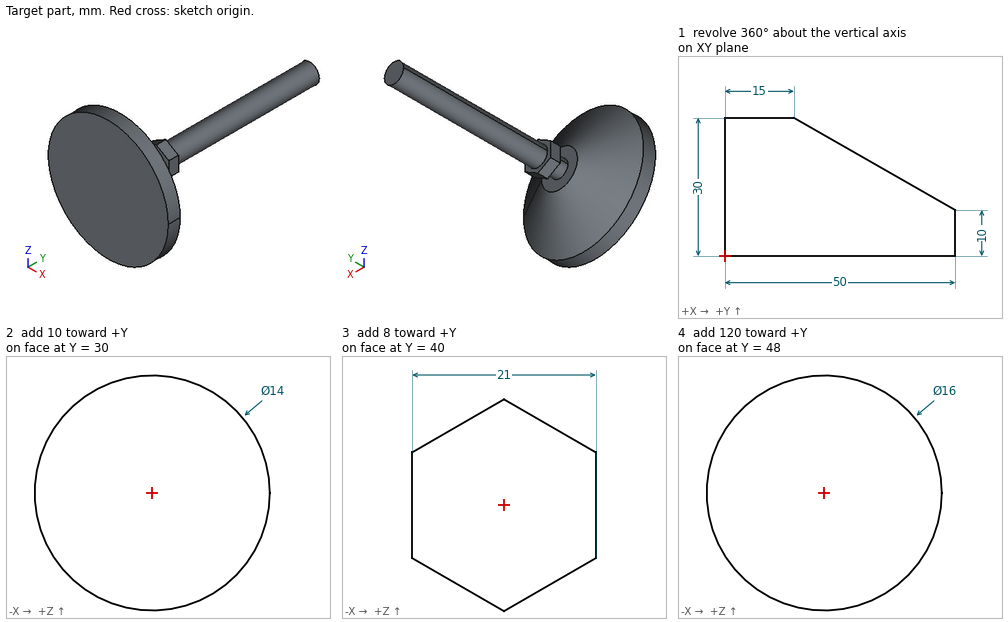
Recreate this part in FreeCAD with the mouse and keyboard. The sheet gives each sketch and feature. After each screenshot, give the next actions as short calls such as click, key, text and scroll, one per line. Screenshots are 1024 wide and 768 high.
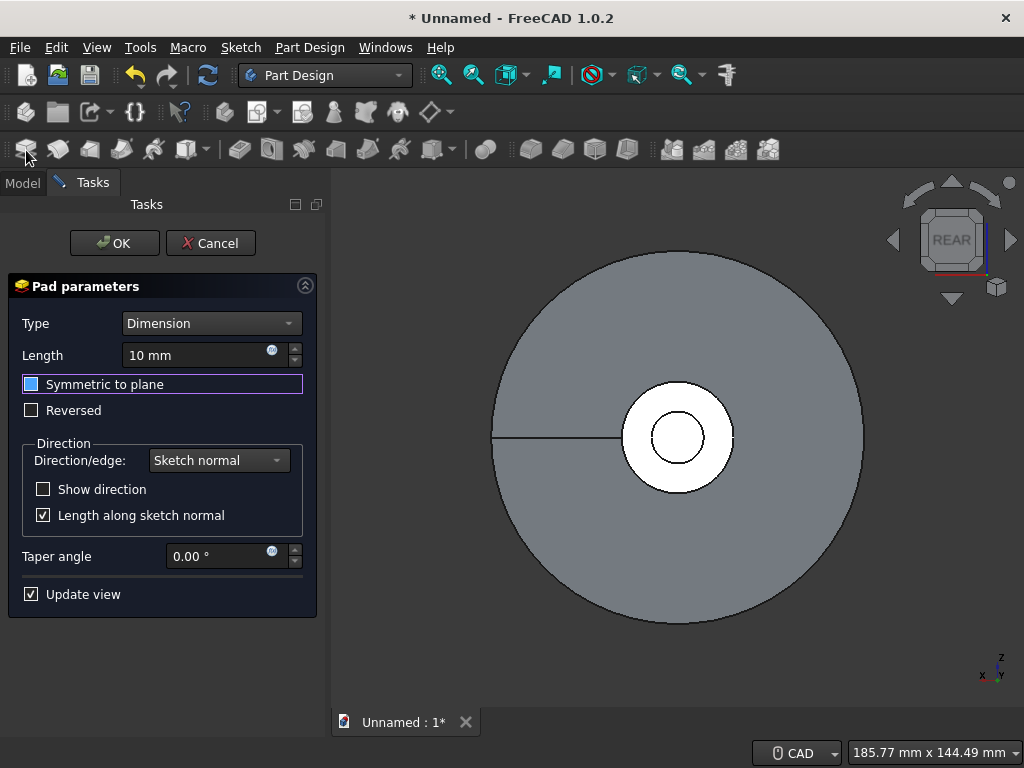
click(115, 243)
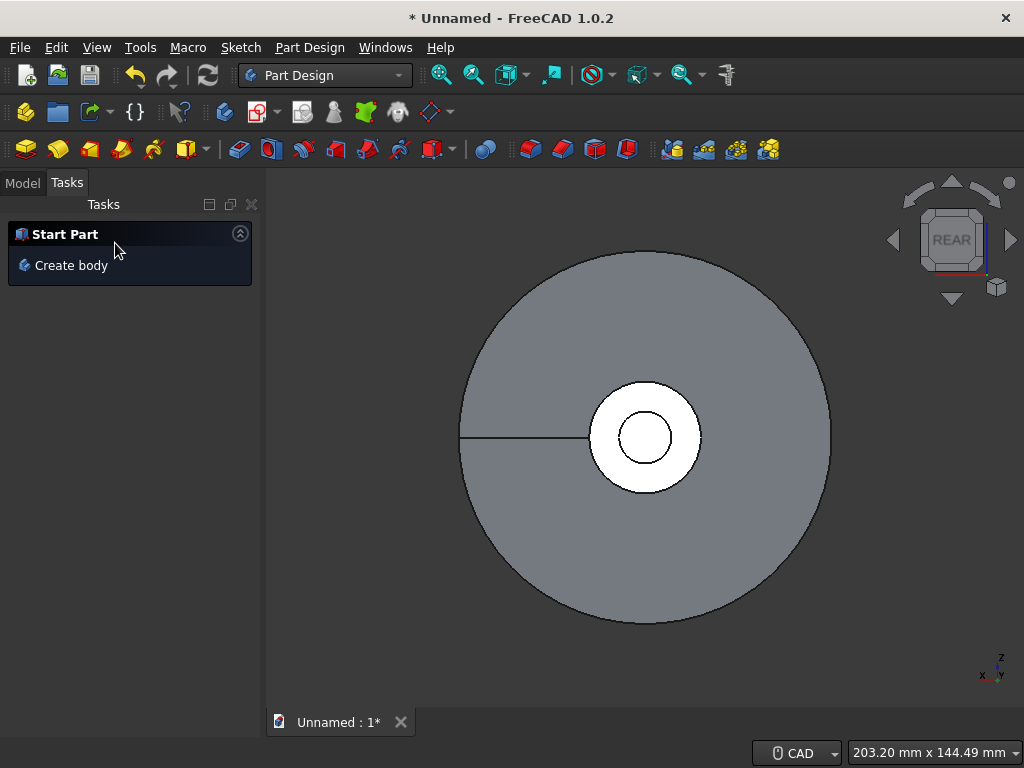
click(645, 436)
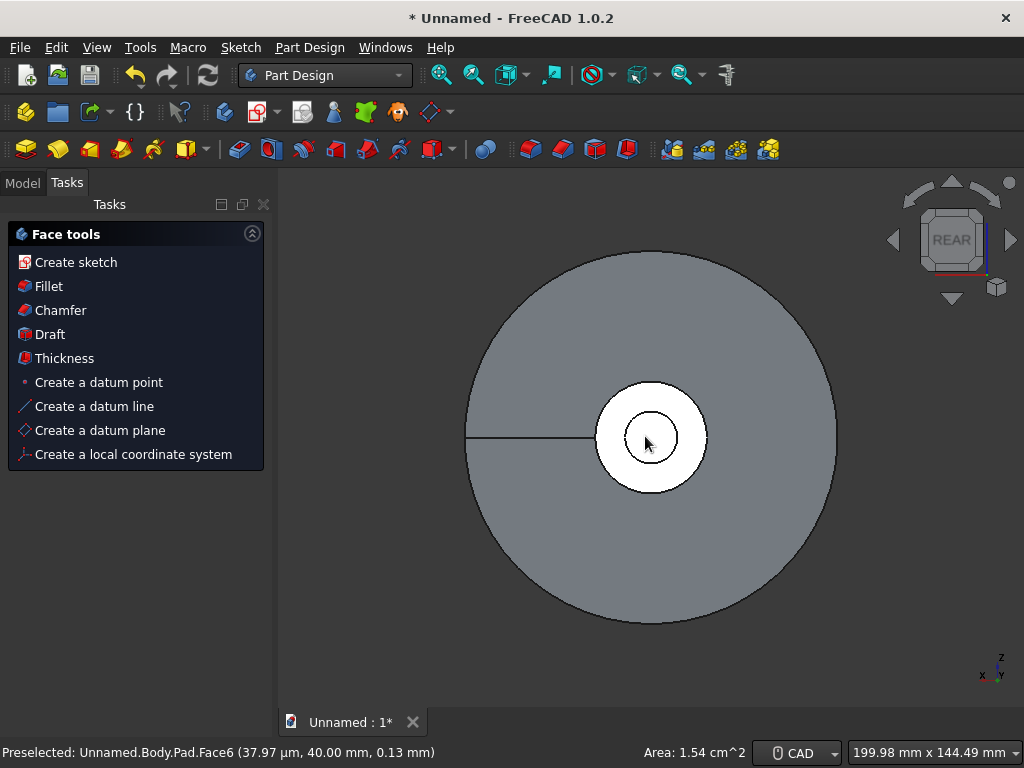
click(258, 112)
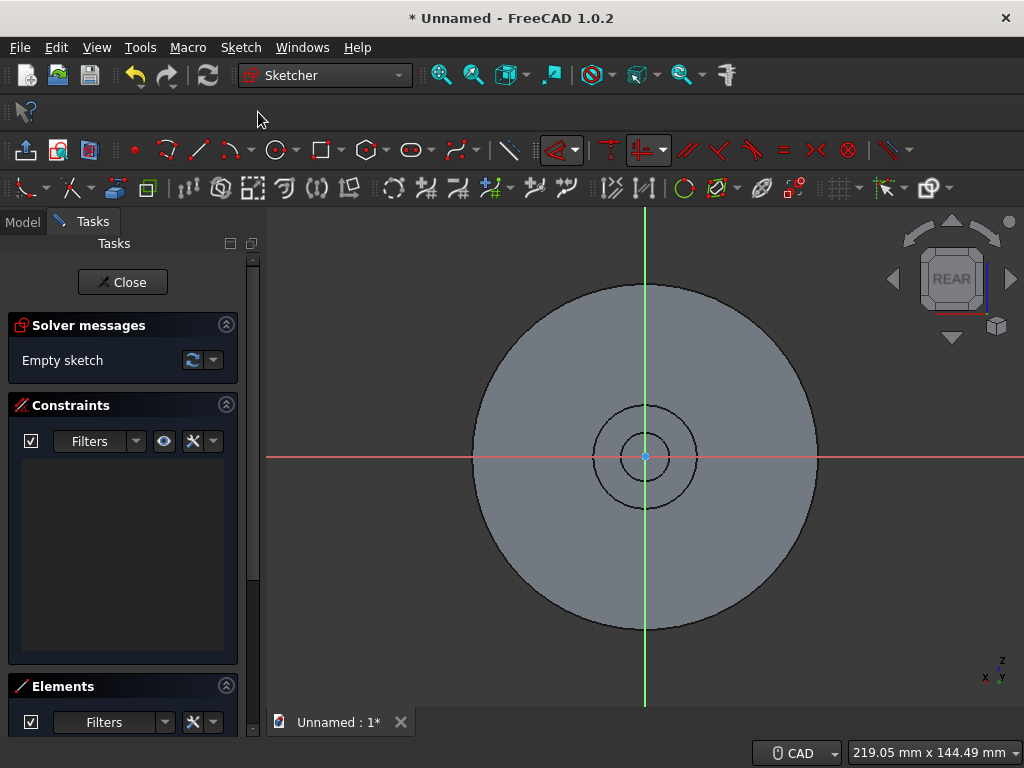
scroll(668, 457, up, 7)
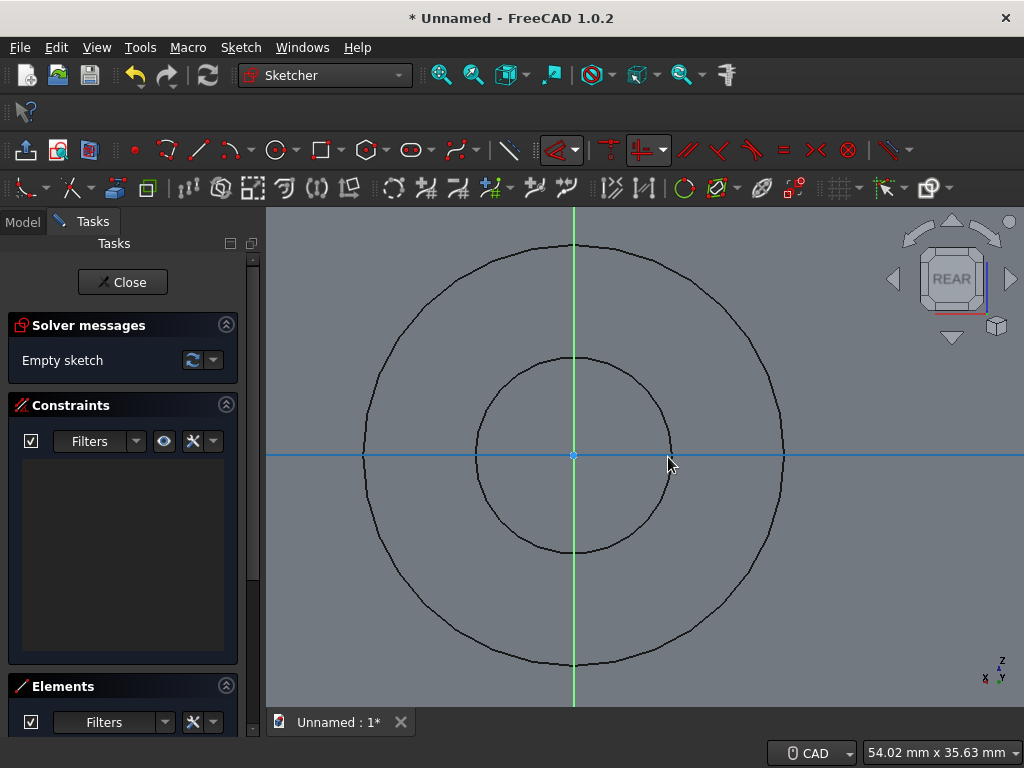
click(366, 150)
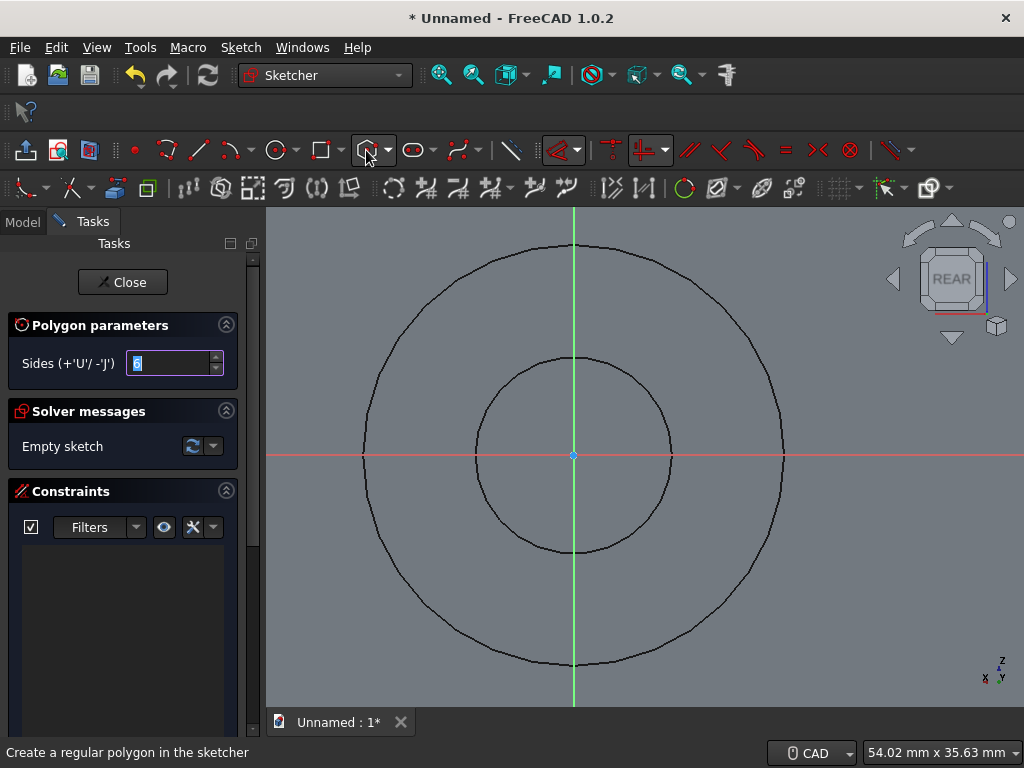
click(574, 455)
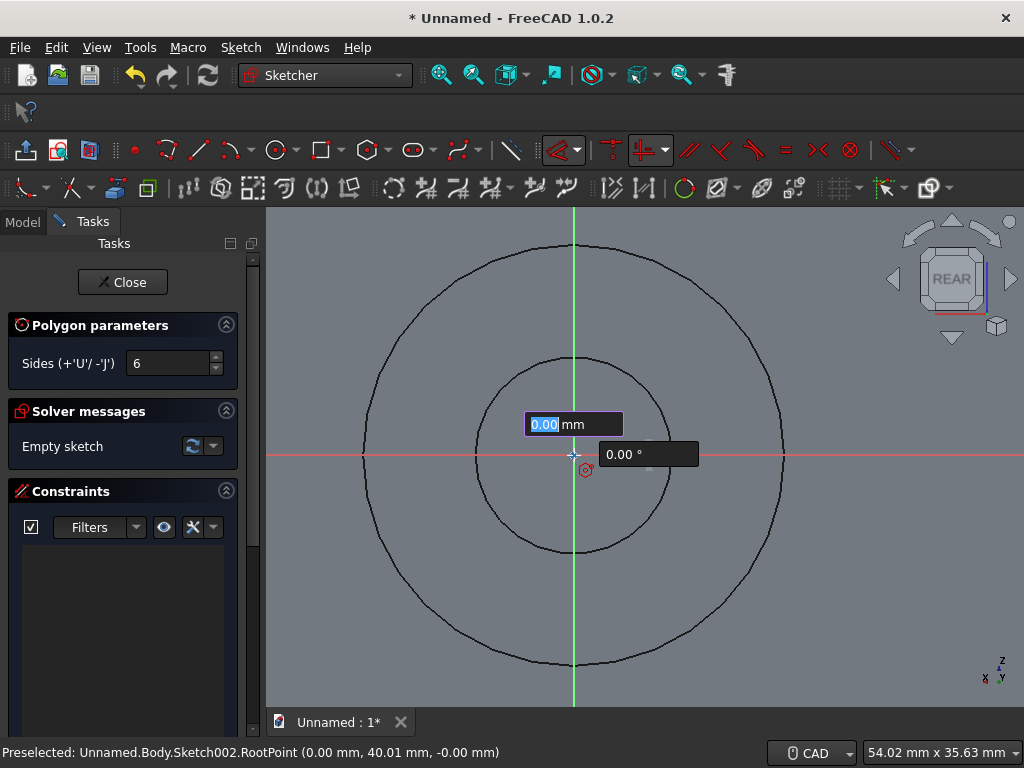
click(574, 626)
key(Escape)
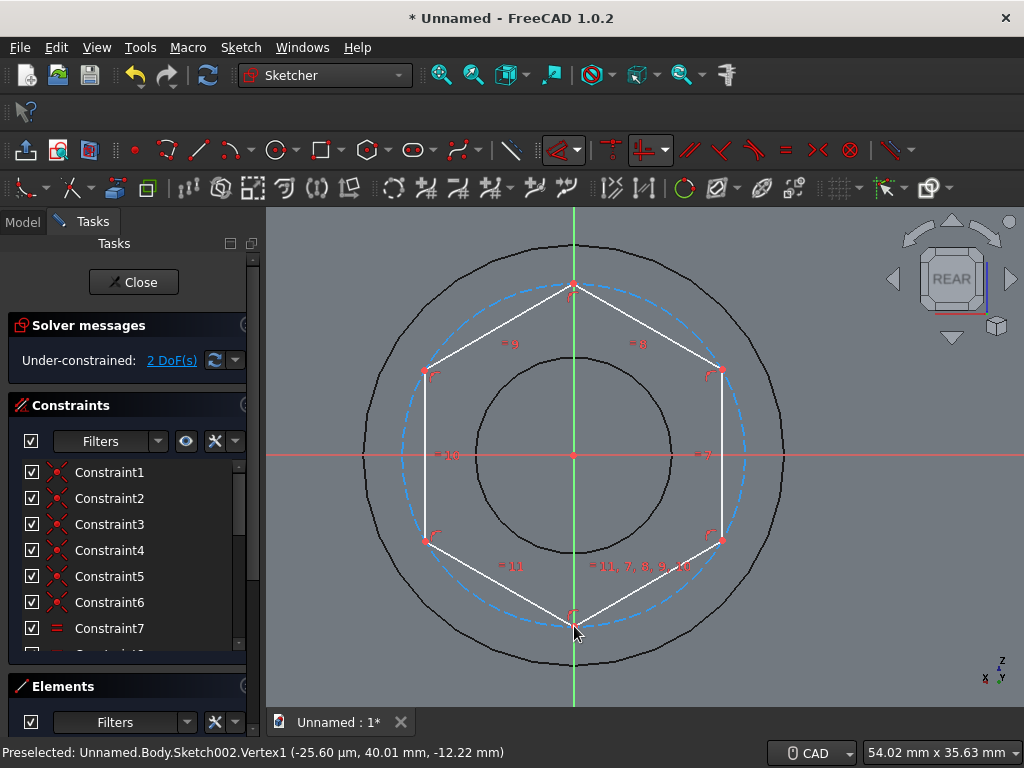
click(722, 489)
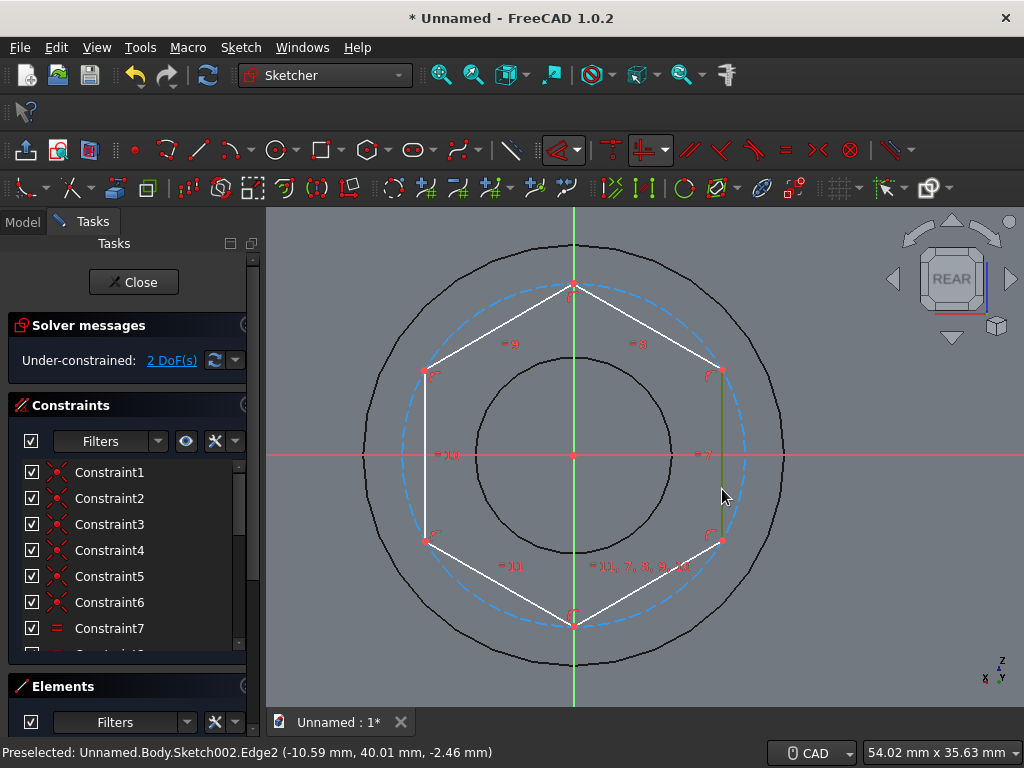
key(v)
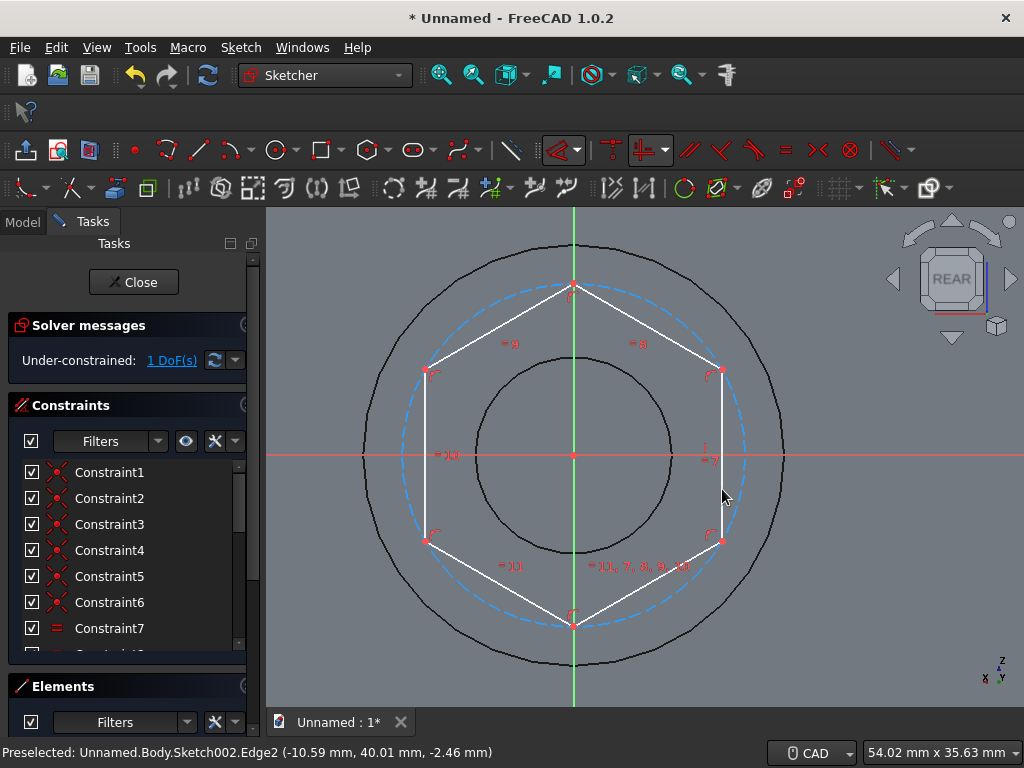
click(425, 370)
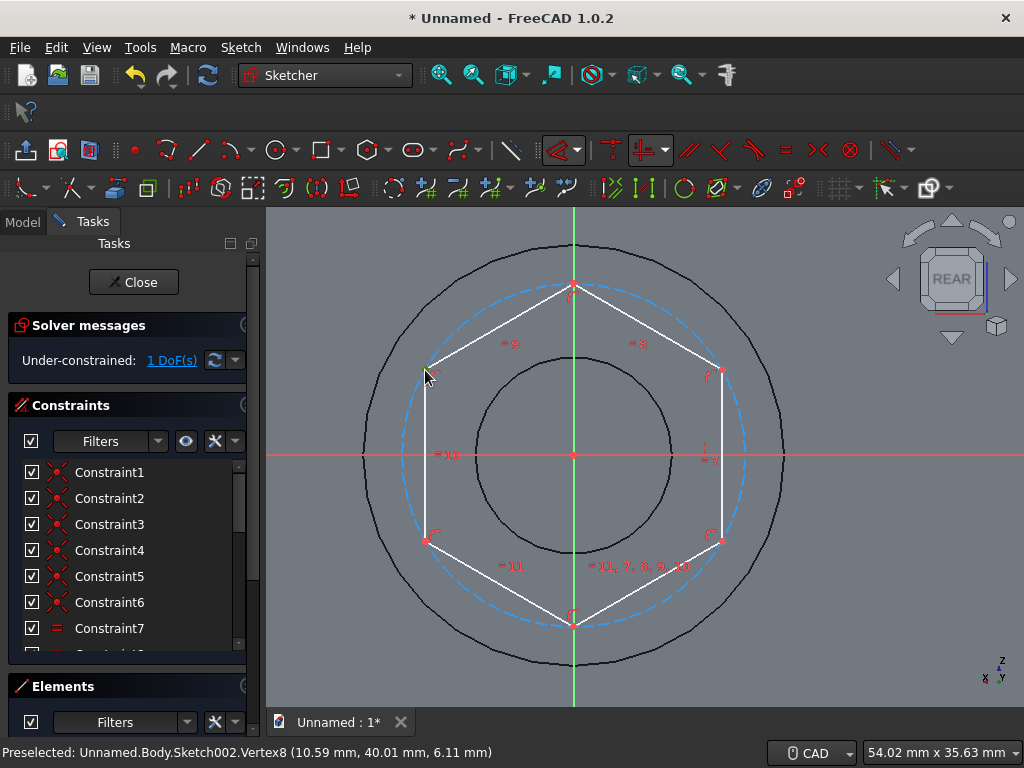
click(722, 541)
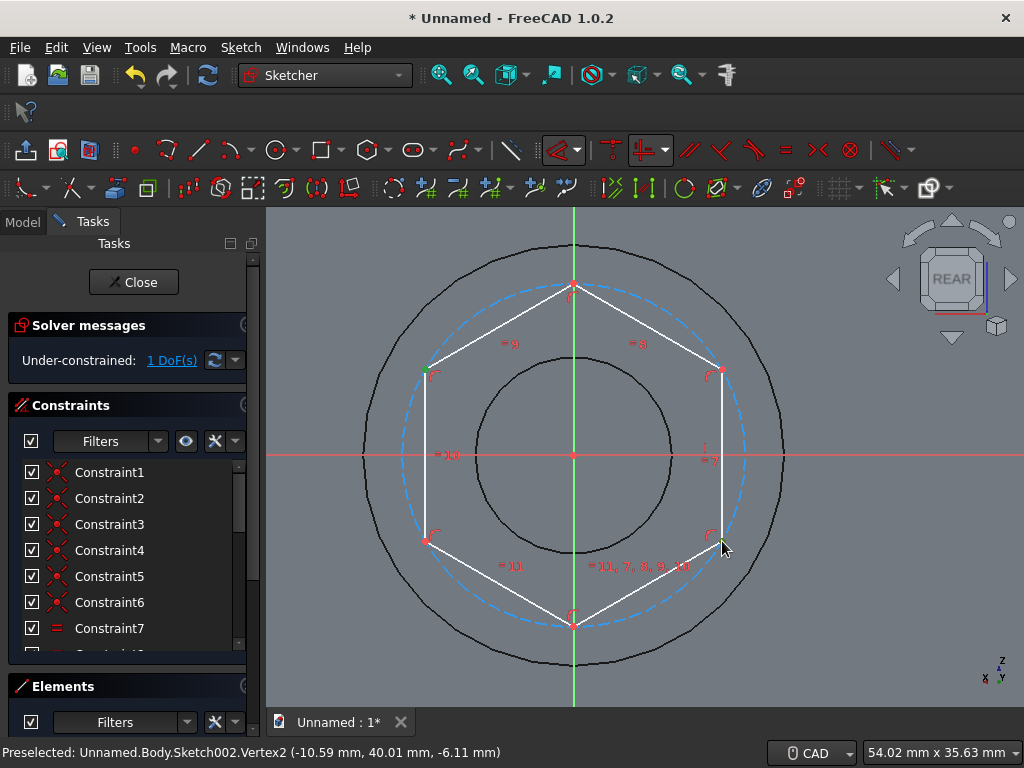
click(580, 150)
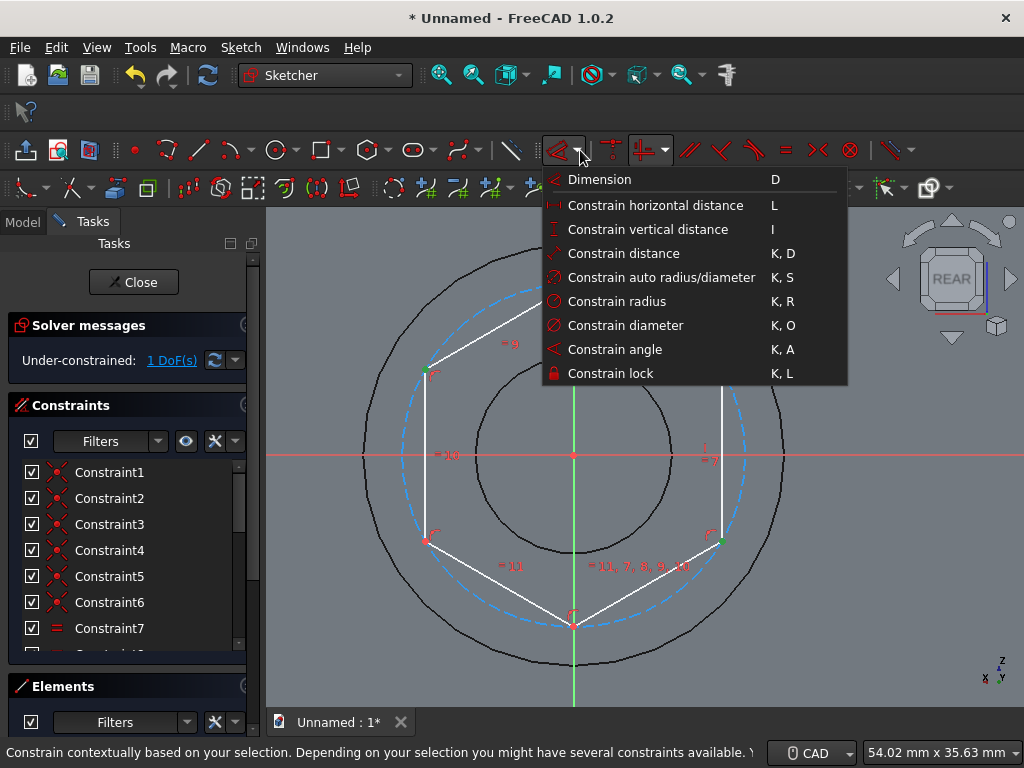
click(695, 205)